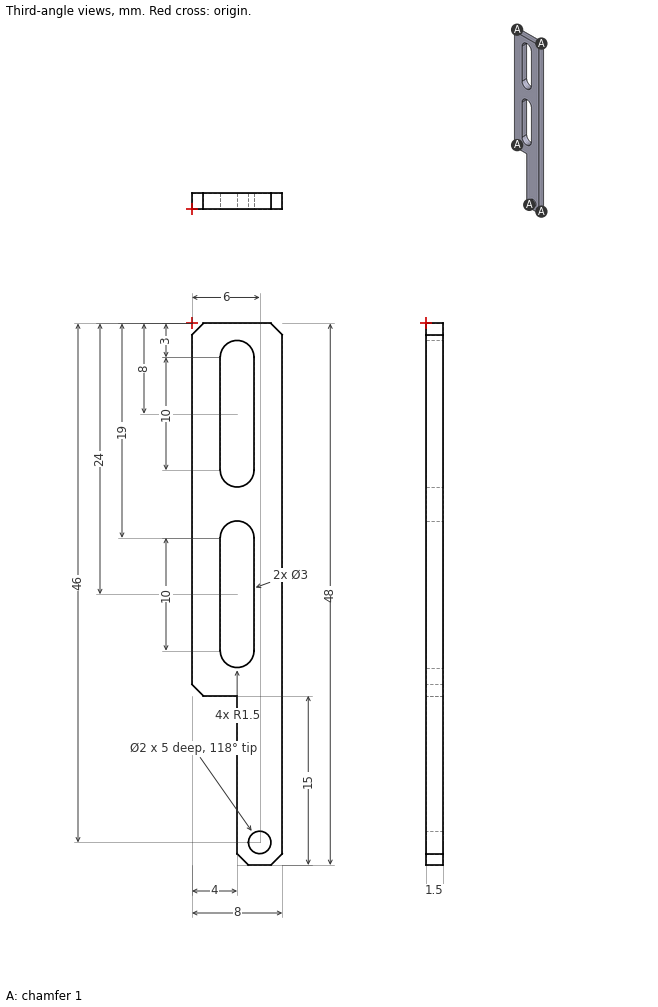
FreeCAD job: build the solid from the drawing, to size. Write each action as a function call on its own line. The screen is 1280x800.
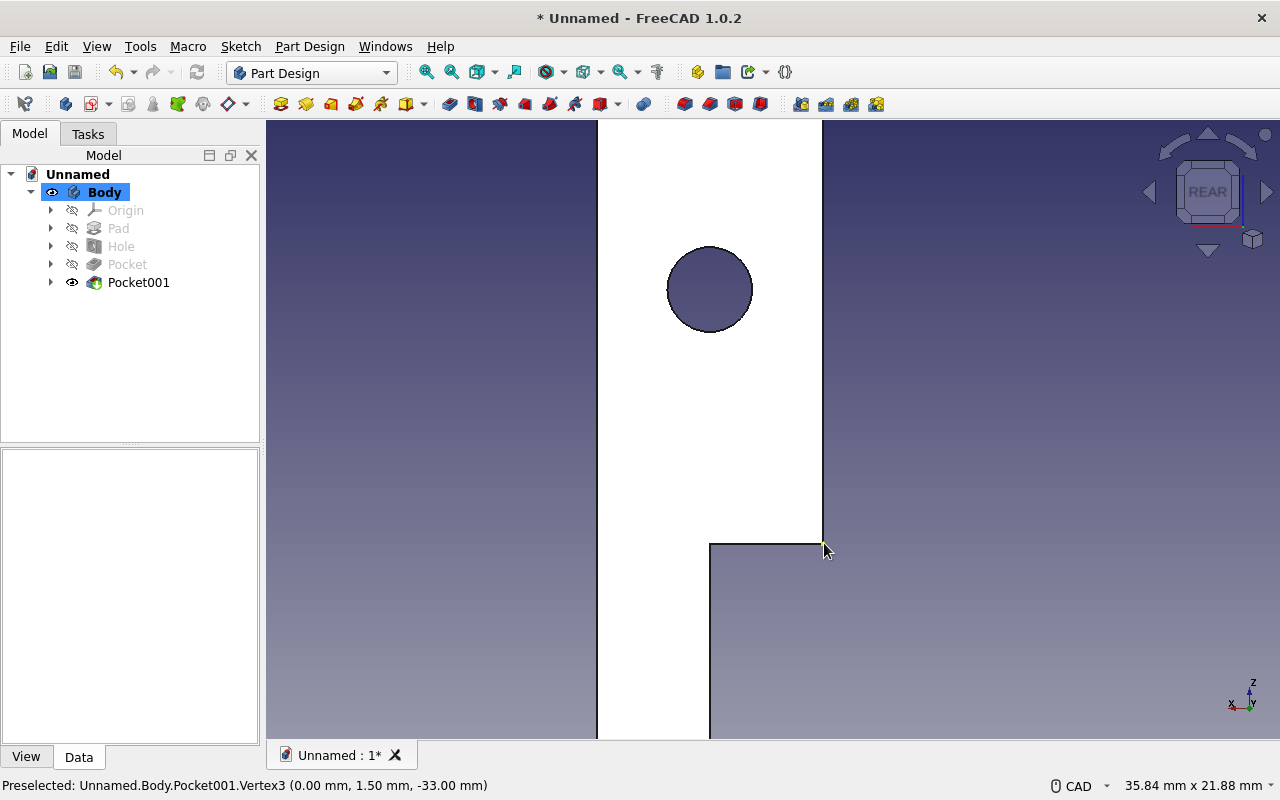
key(v)
key(f)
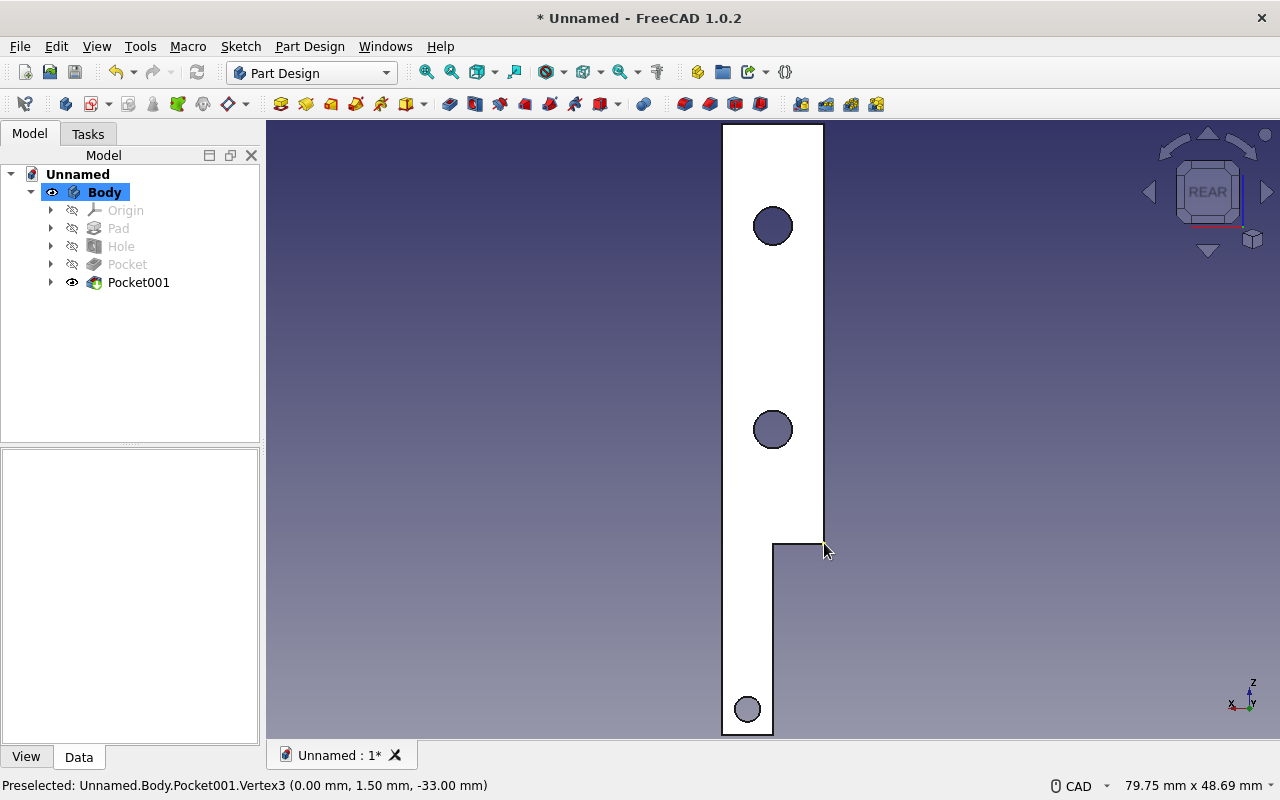
key(0)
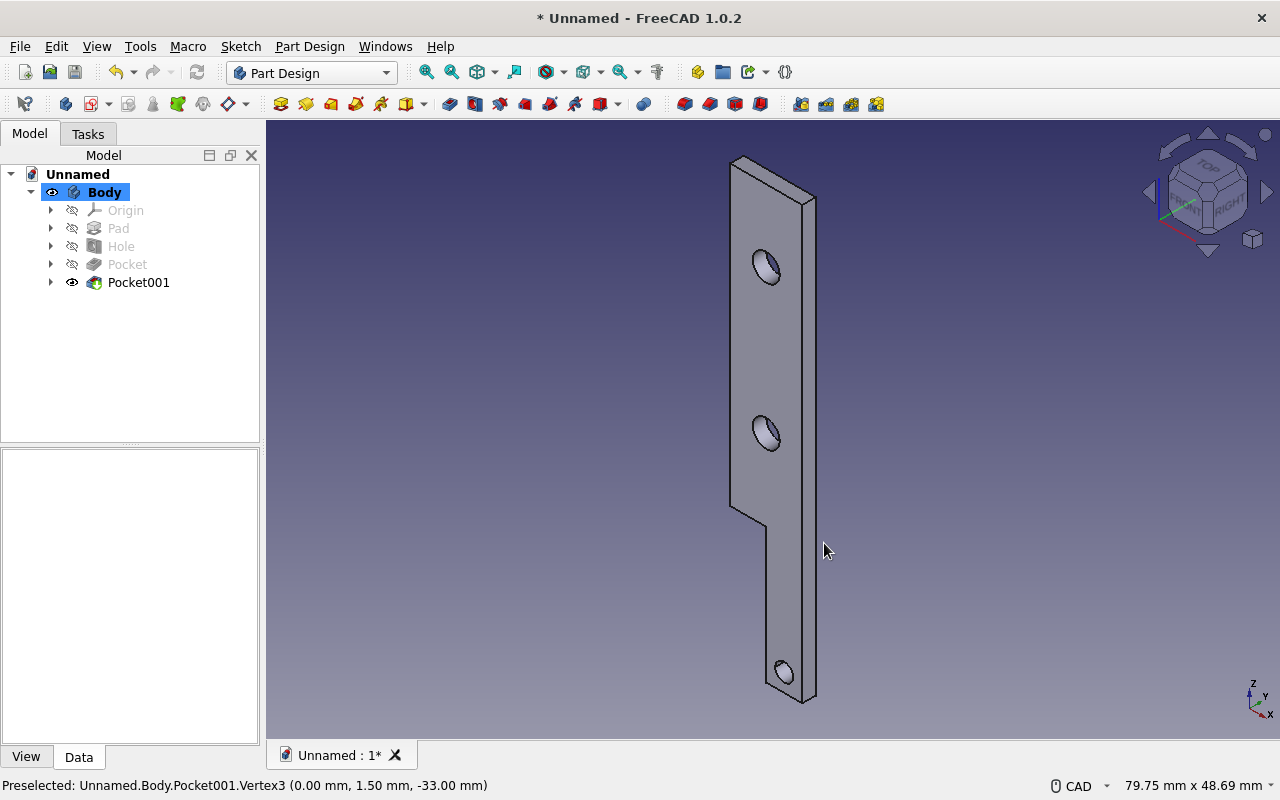
click(809, 200)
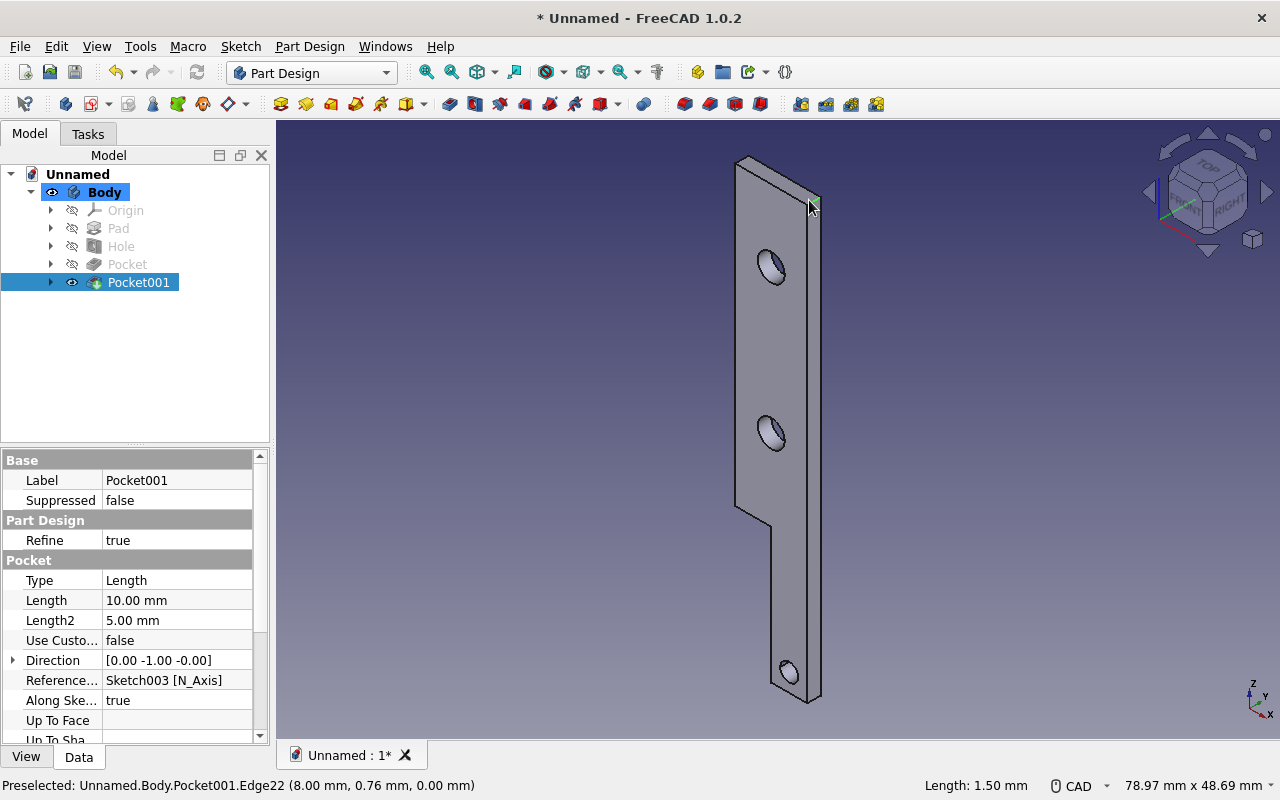
scroll(742, 501, up, 4)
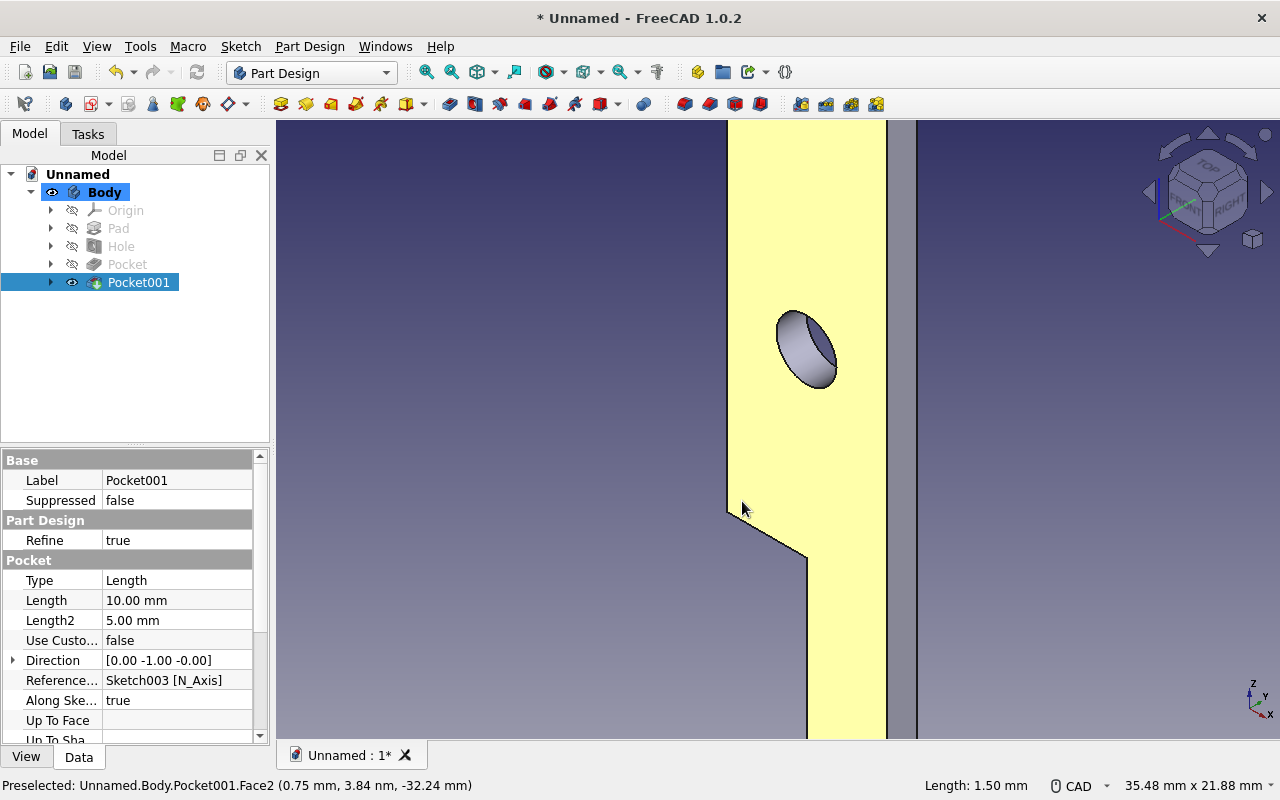
click(427, 72)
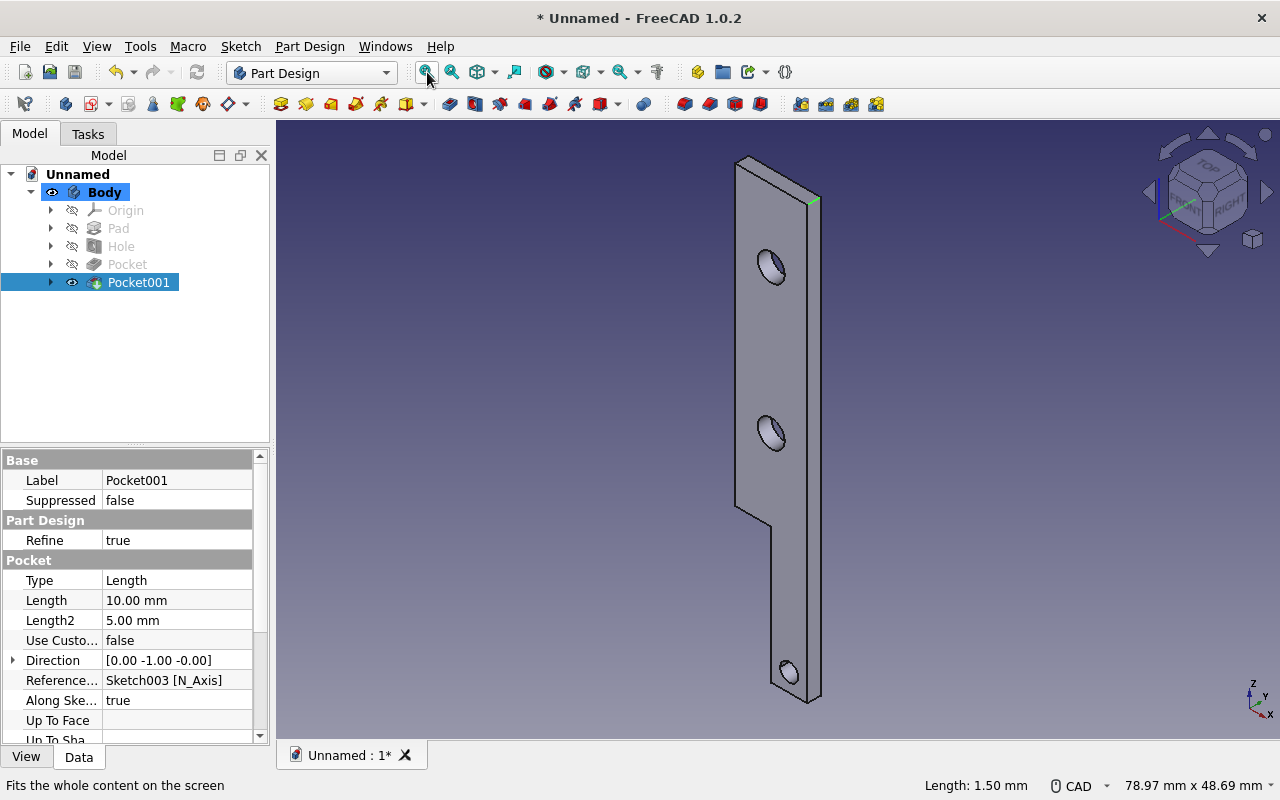
key(2)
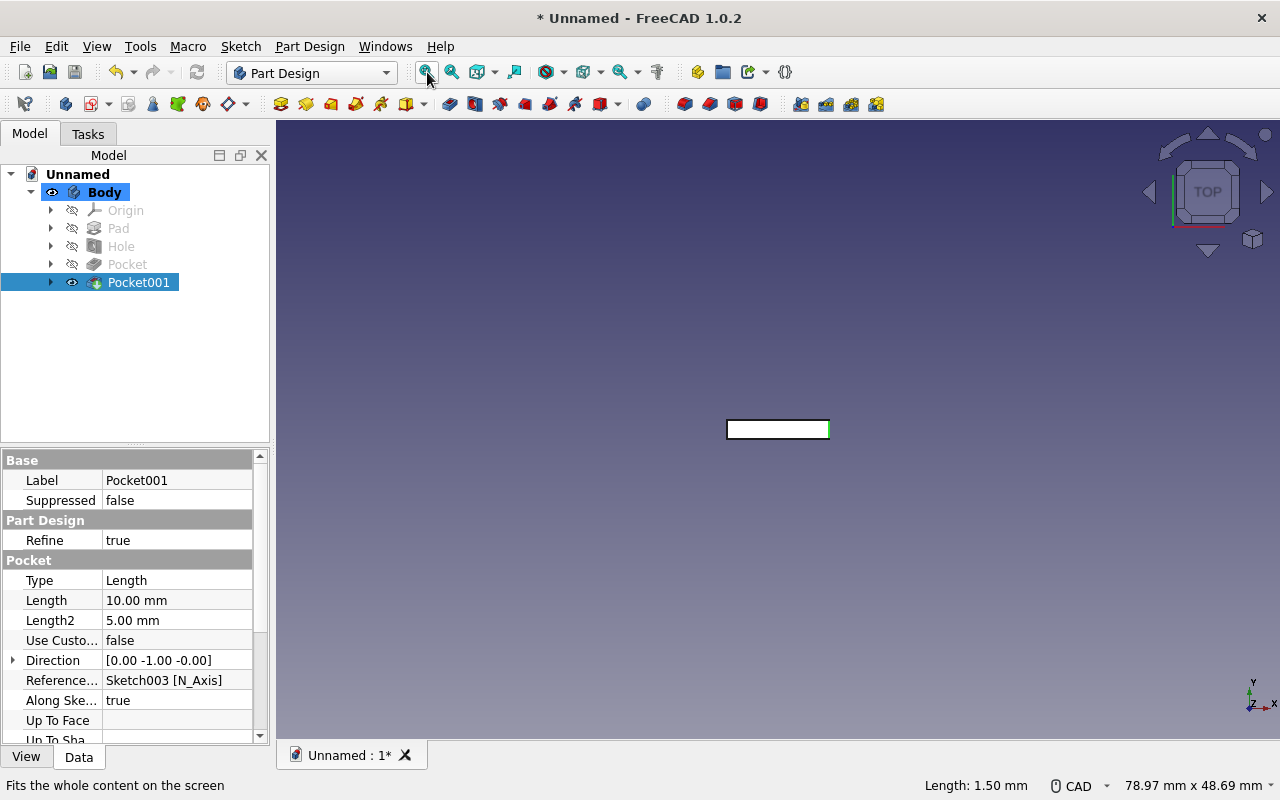
key(v)
key(f)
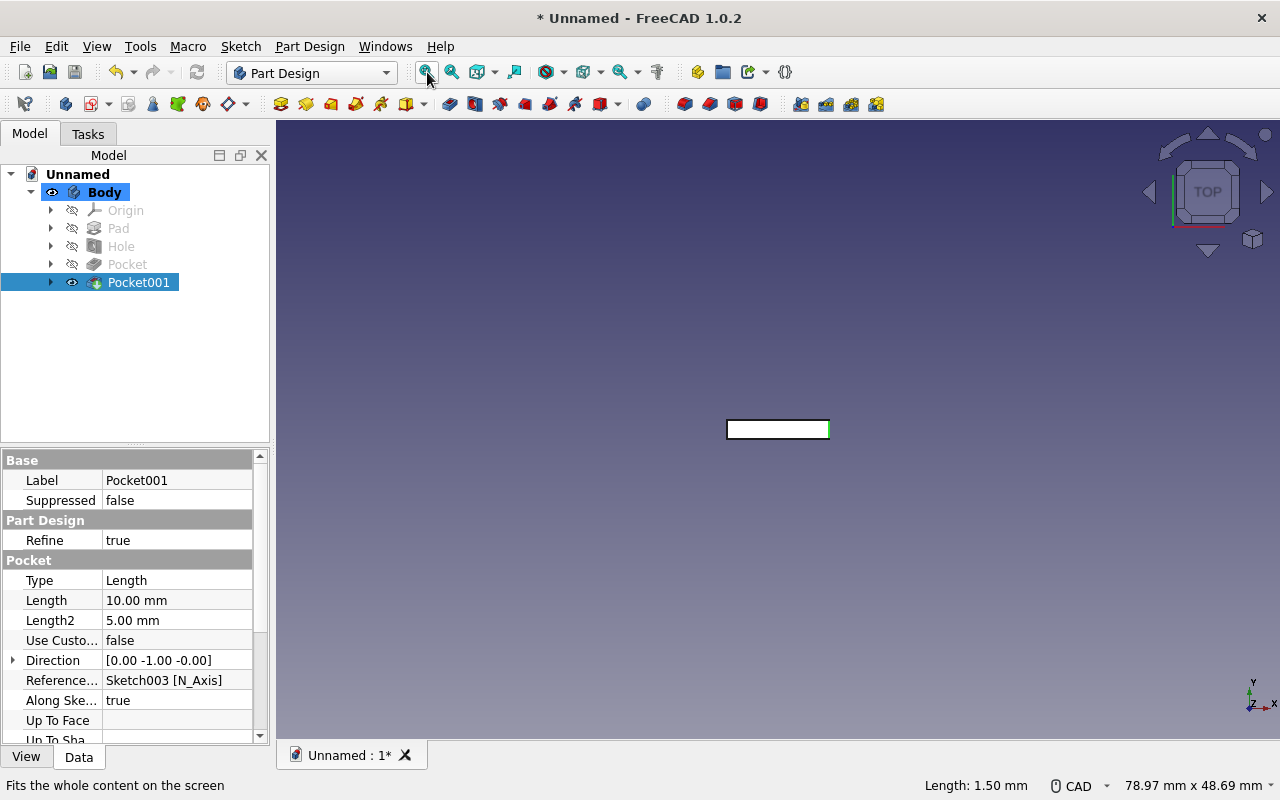
click(727, 429, ctrl)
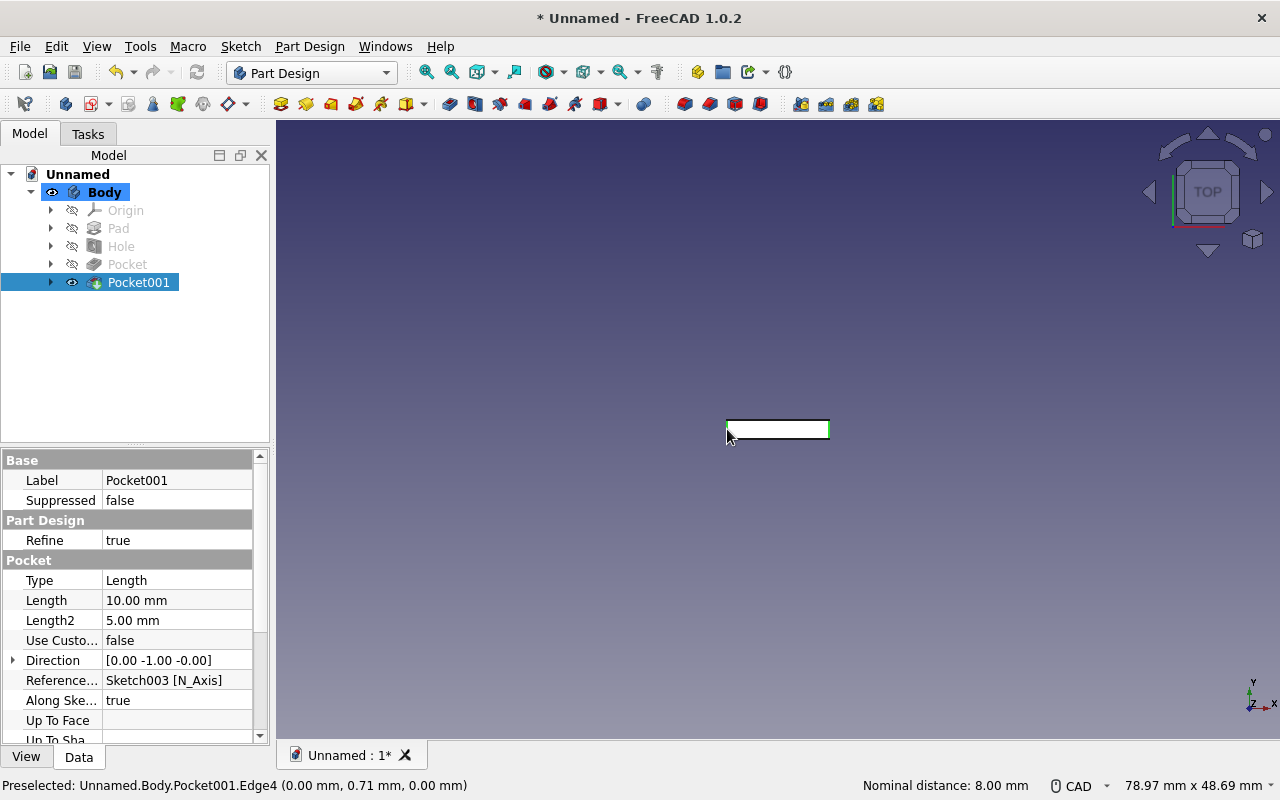
scroll(727, 429, up, 4)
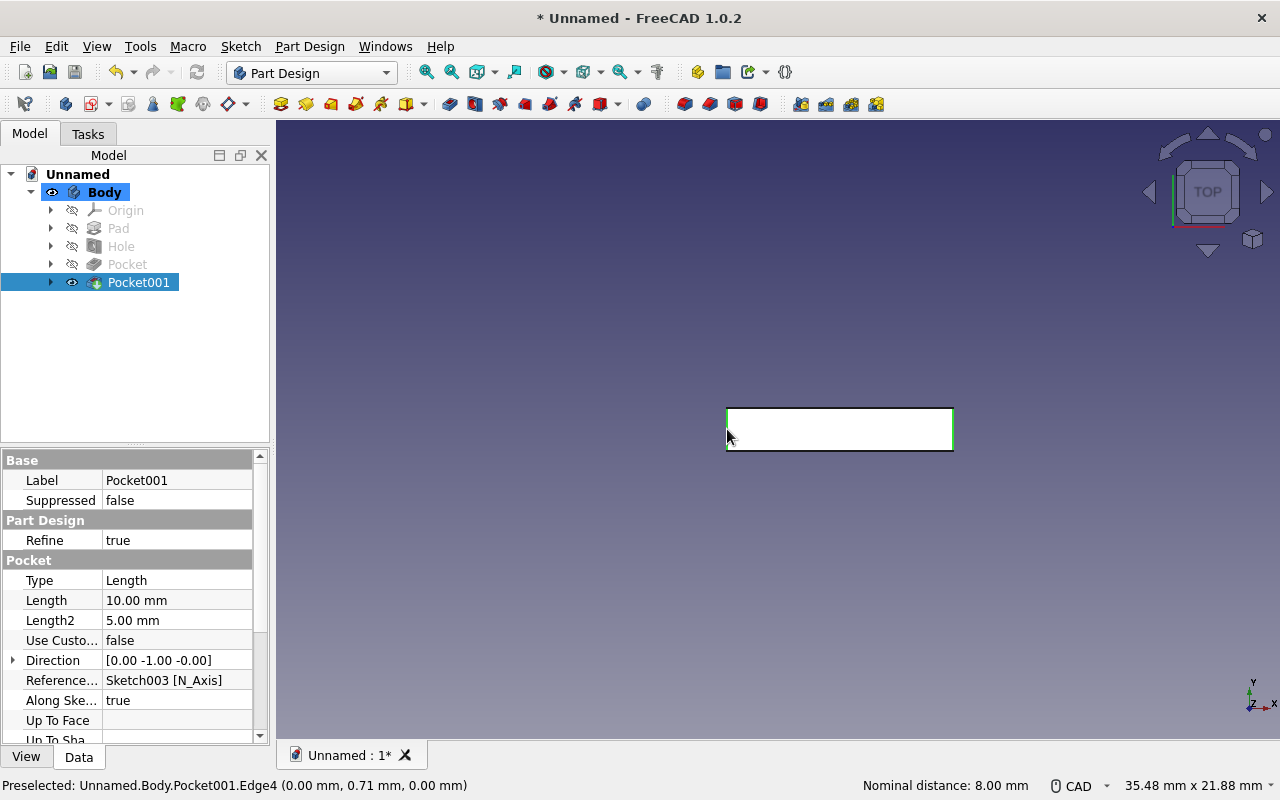
key(v)
key(f)